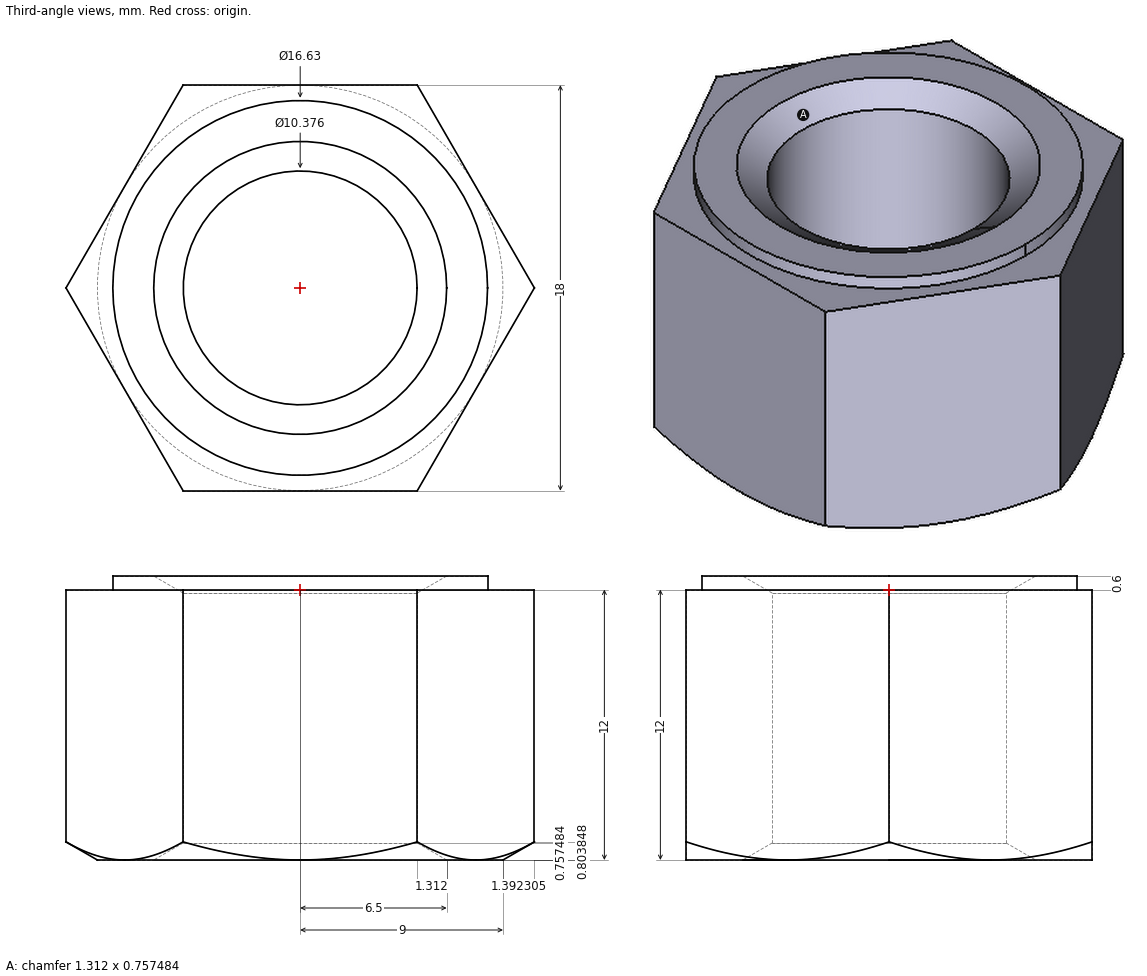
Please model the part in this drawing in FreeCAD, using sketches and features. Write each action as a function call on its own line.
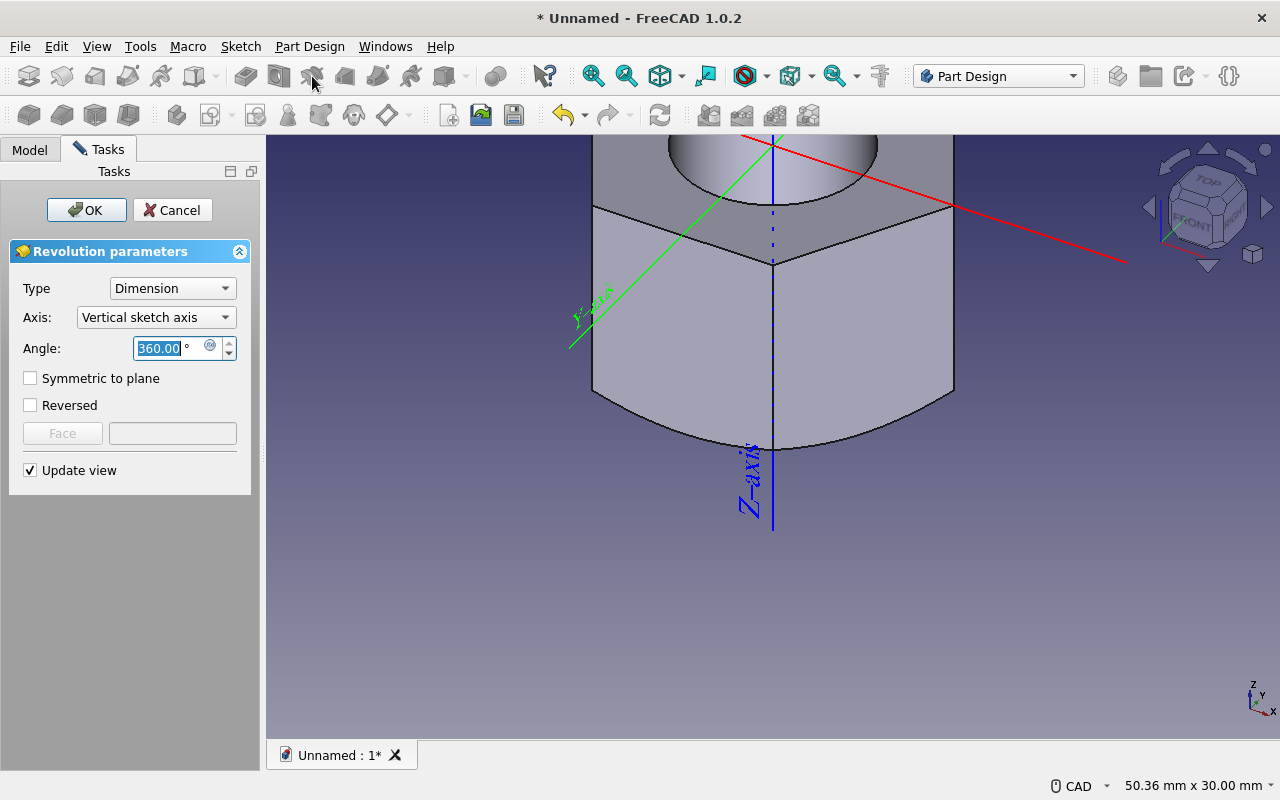
click(87, 210)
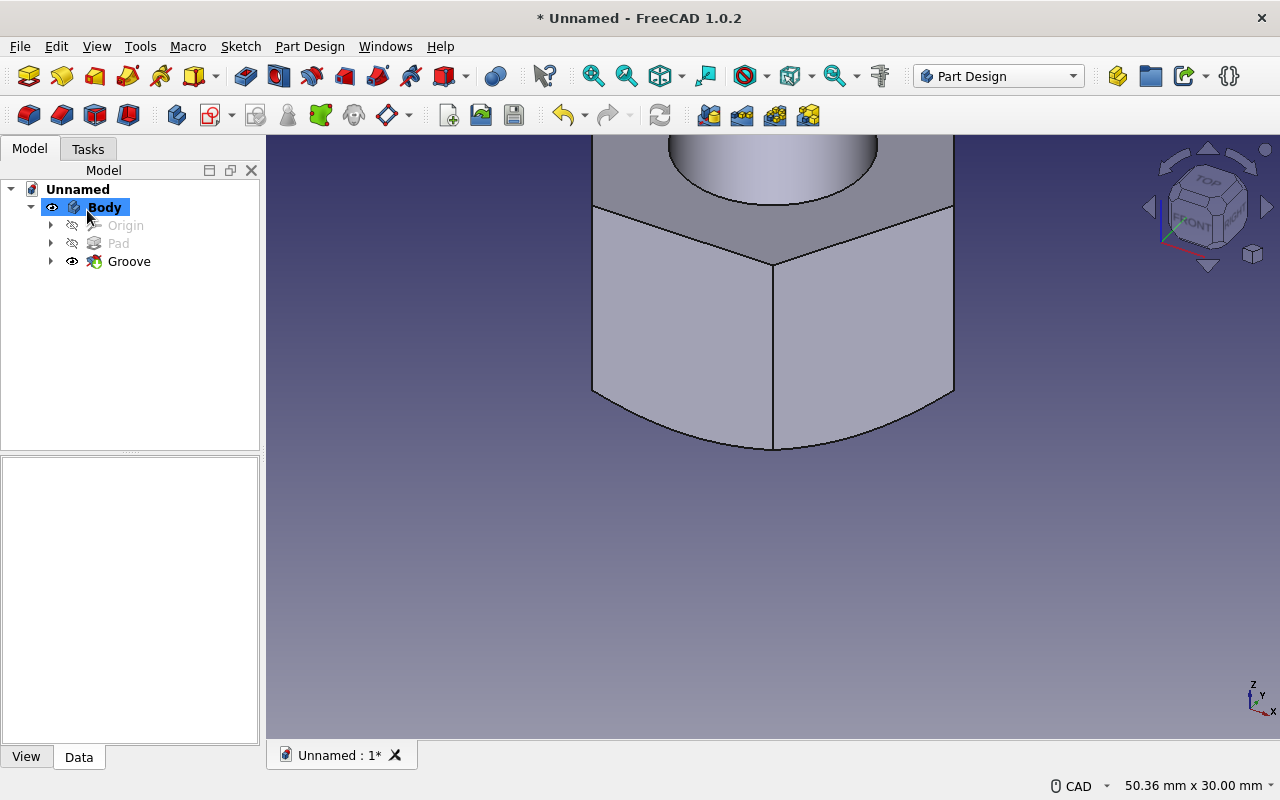
key(v)
key(f)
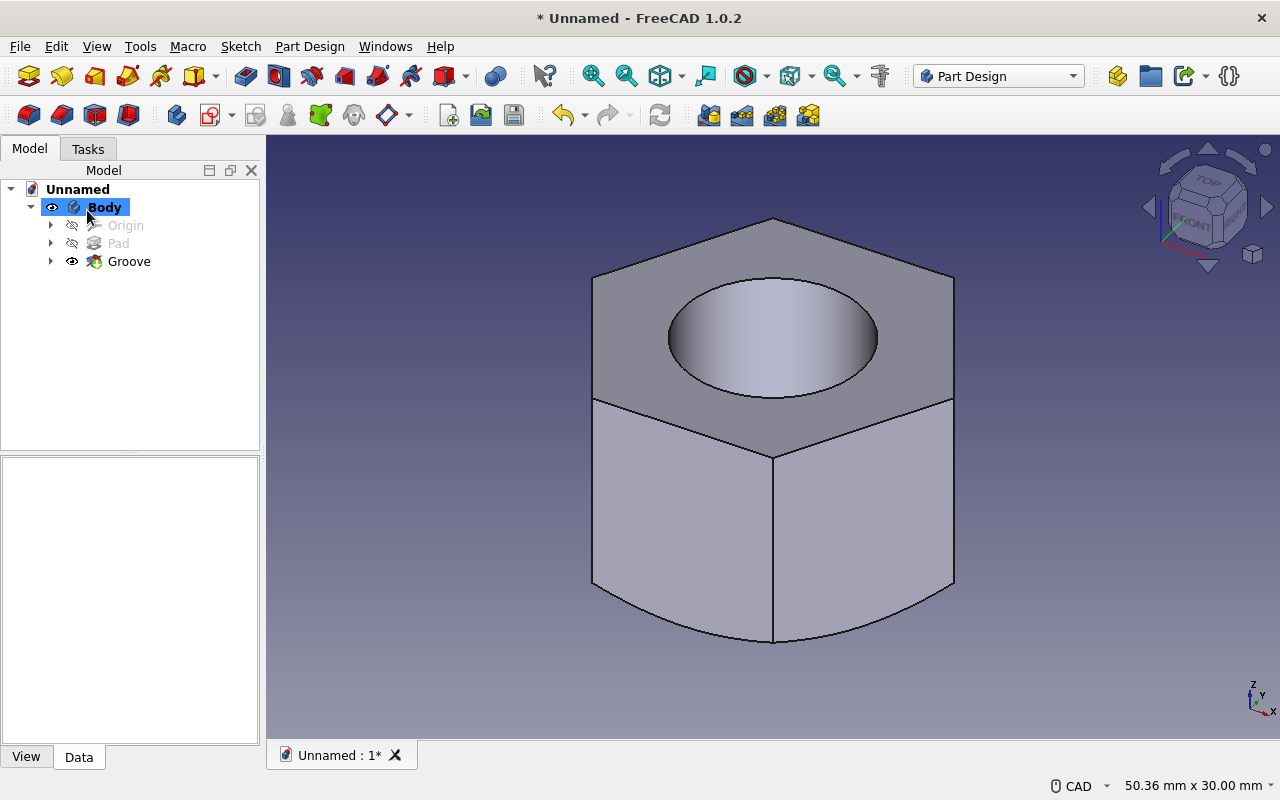
click(210, 116)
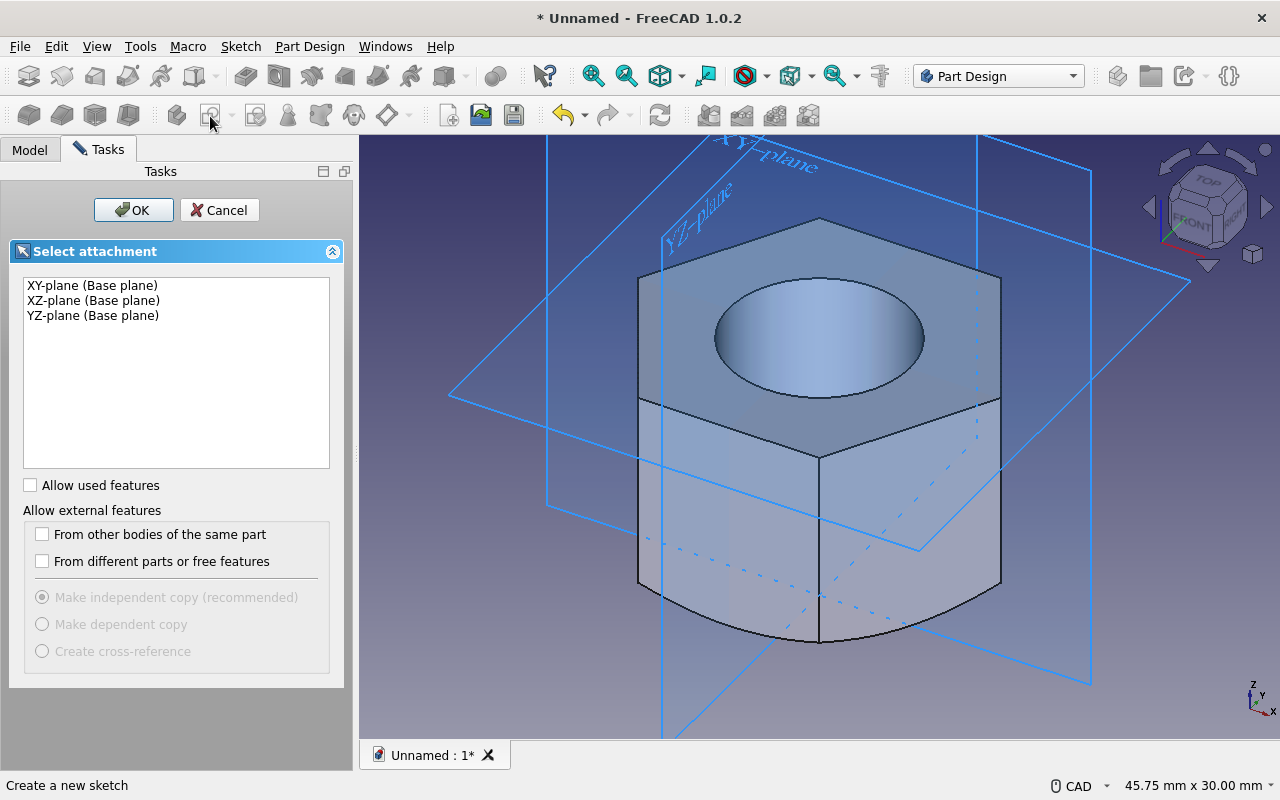
click(84, 300)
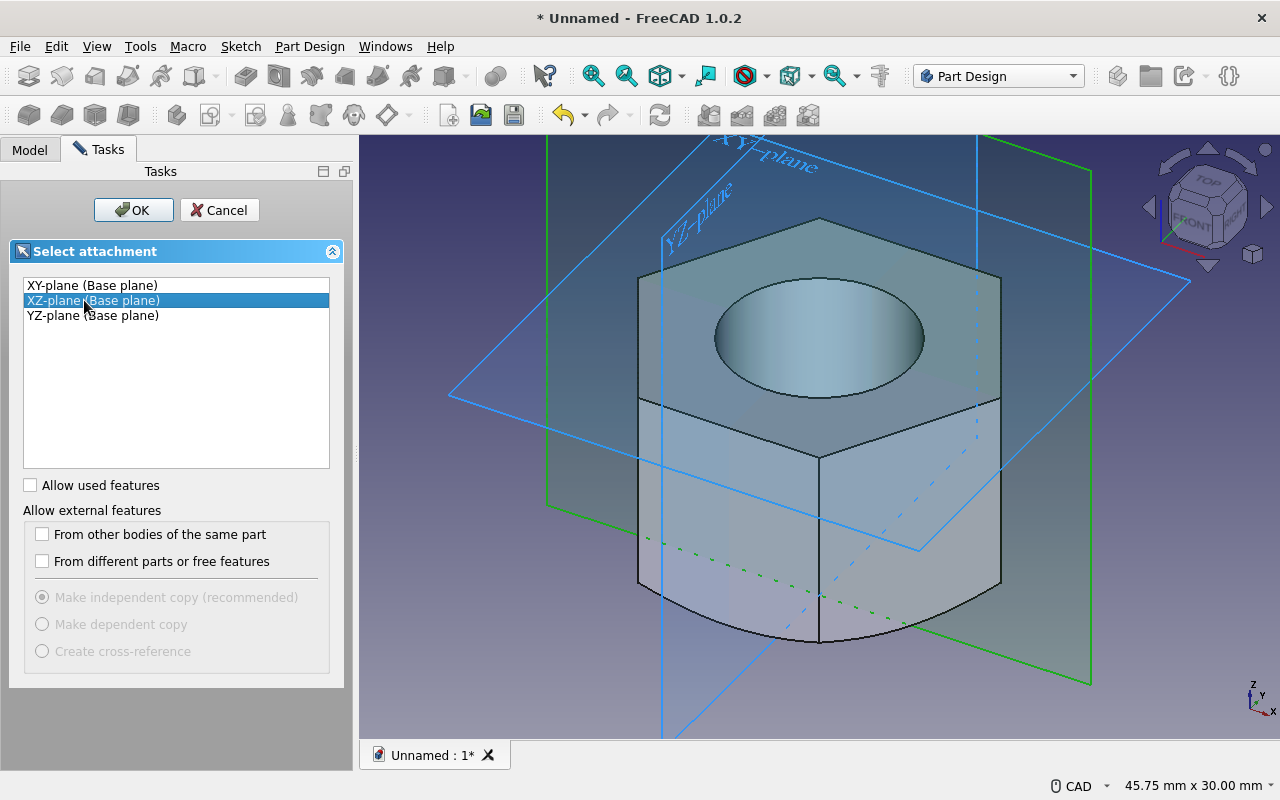
click(134, 210)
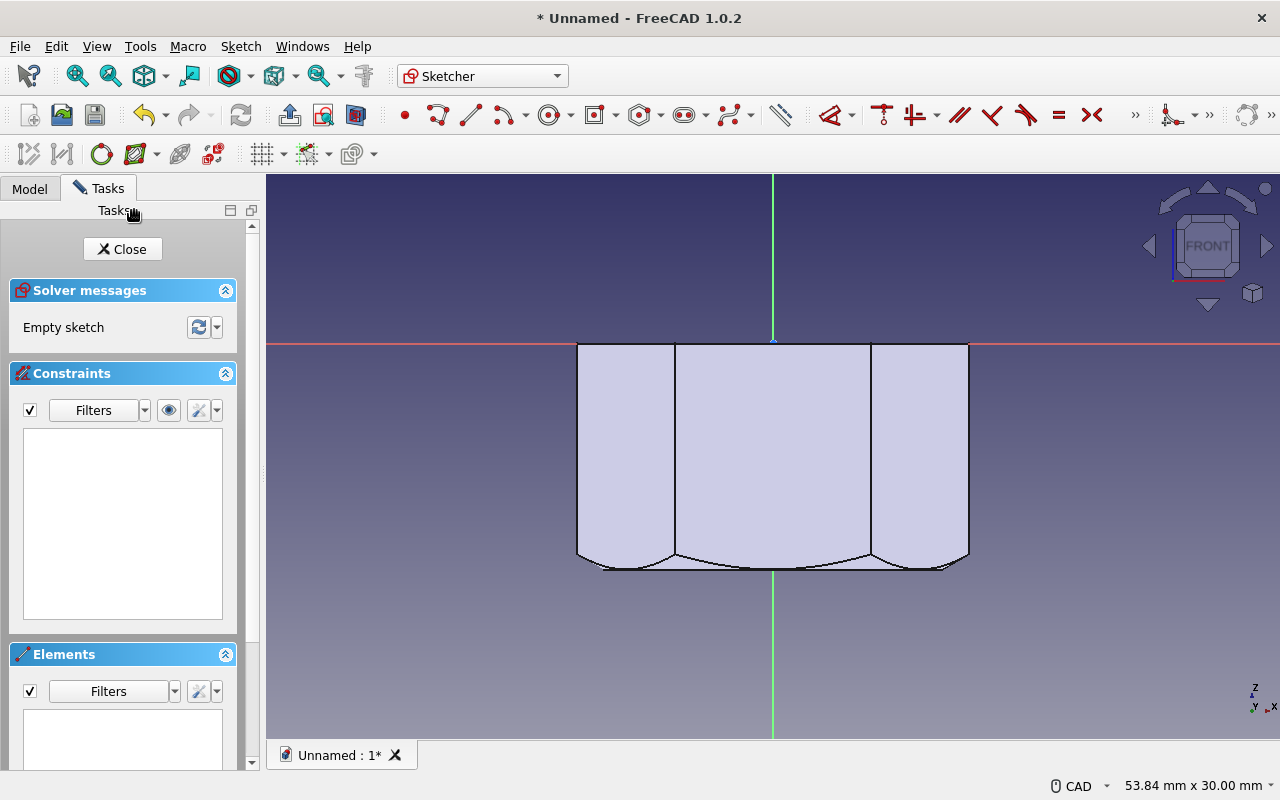
key(q)
key(s)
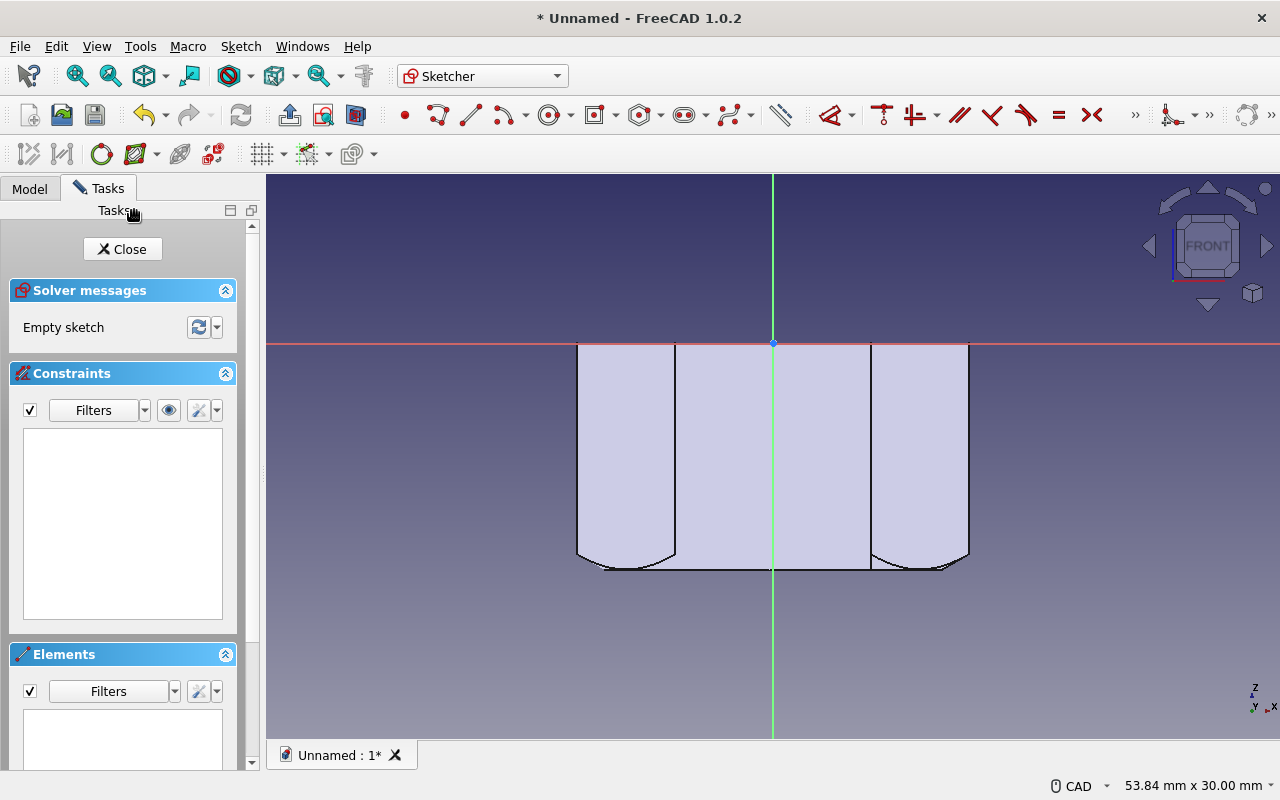
scroll(892, 568, up, 15)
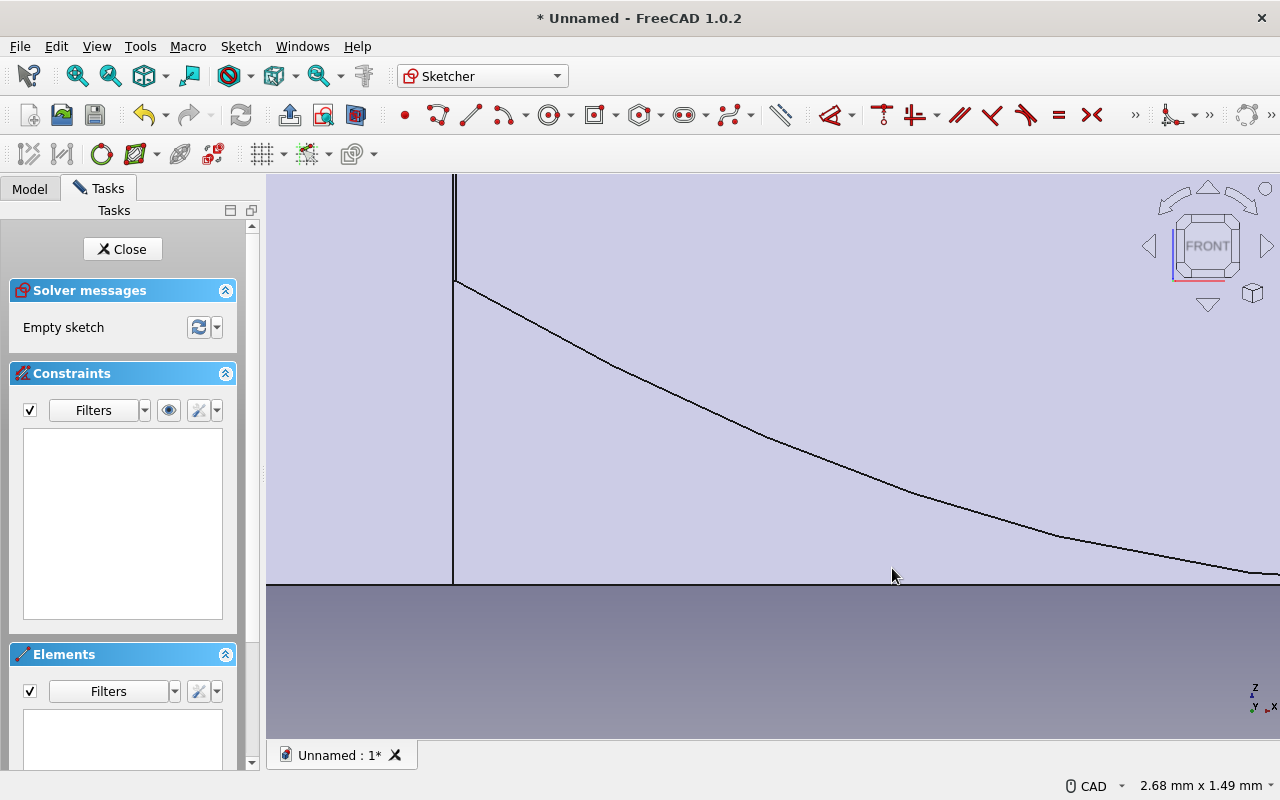
key(g)
key(m)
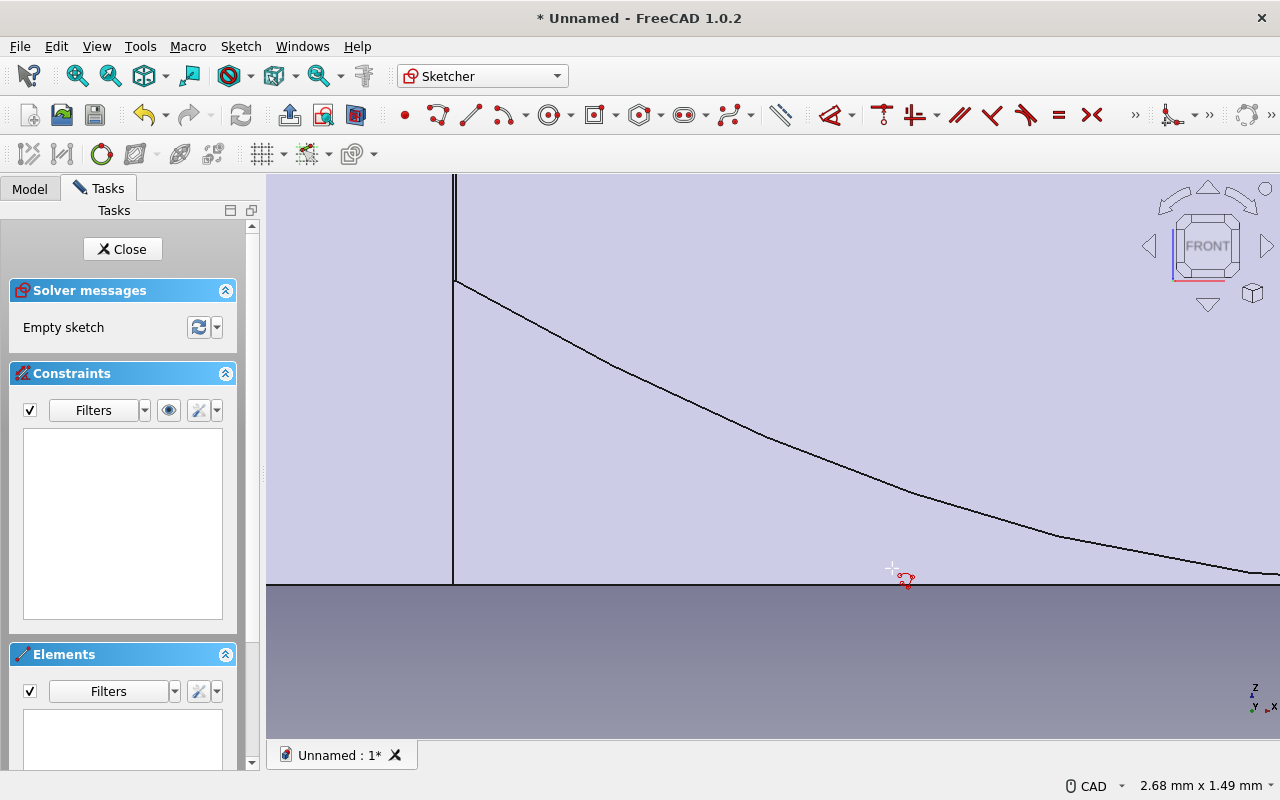
click(453, 298)
click(949, 585)
click(453, 585)
click(453, 299)
key(Escape)
key(Escape)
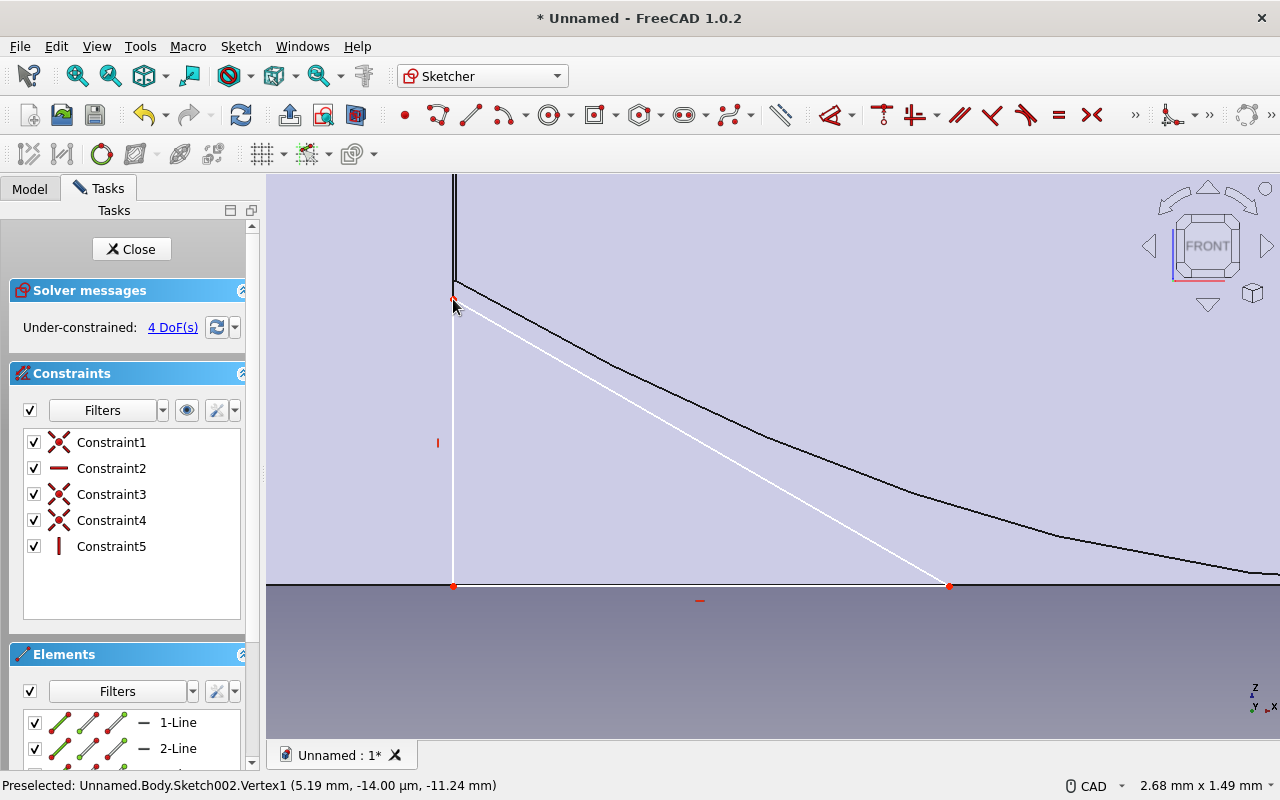
click(830, 116)